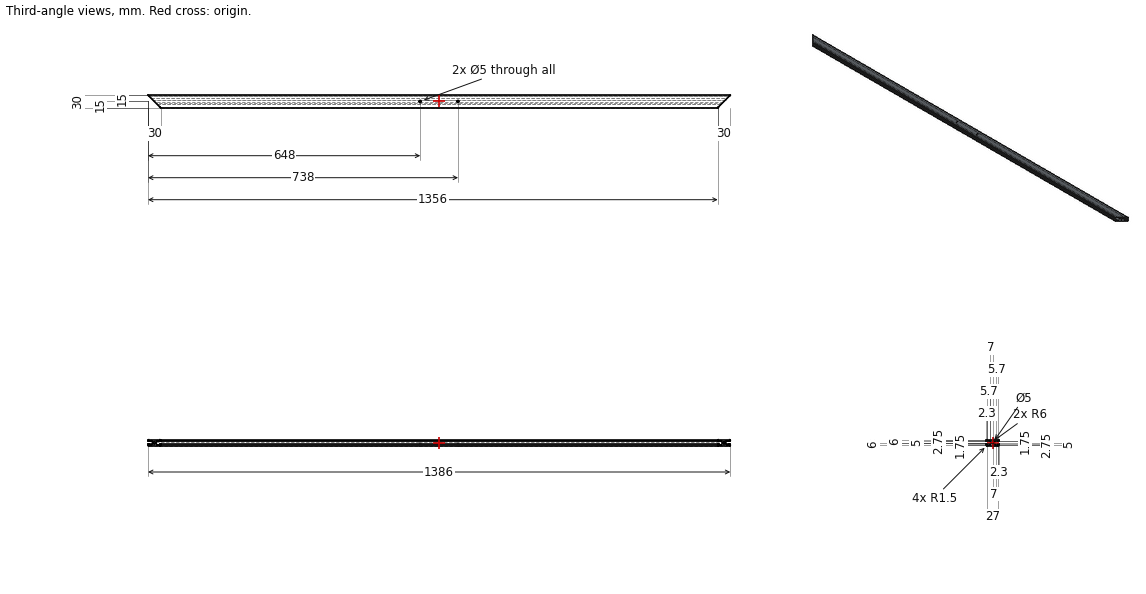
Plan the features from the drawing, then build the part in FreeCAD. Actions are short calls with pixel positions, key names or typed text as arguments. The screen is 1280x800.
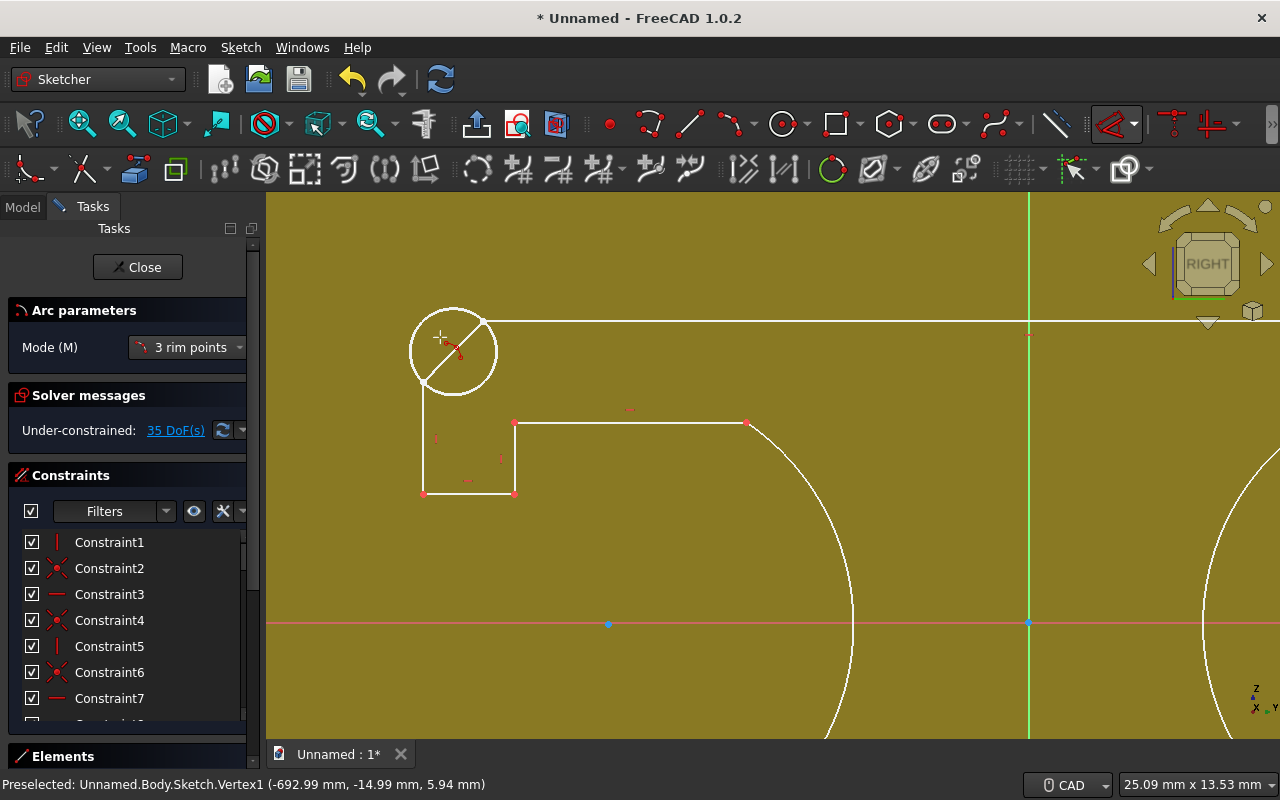
click(440, 337)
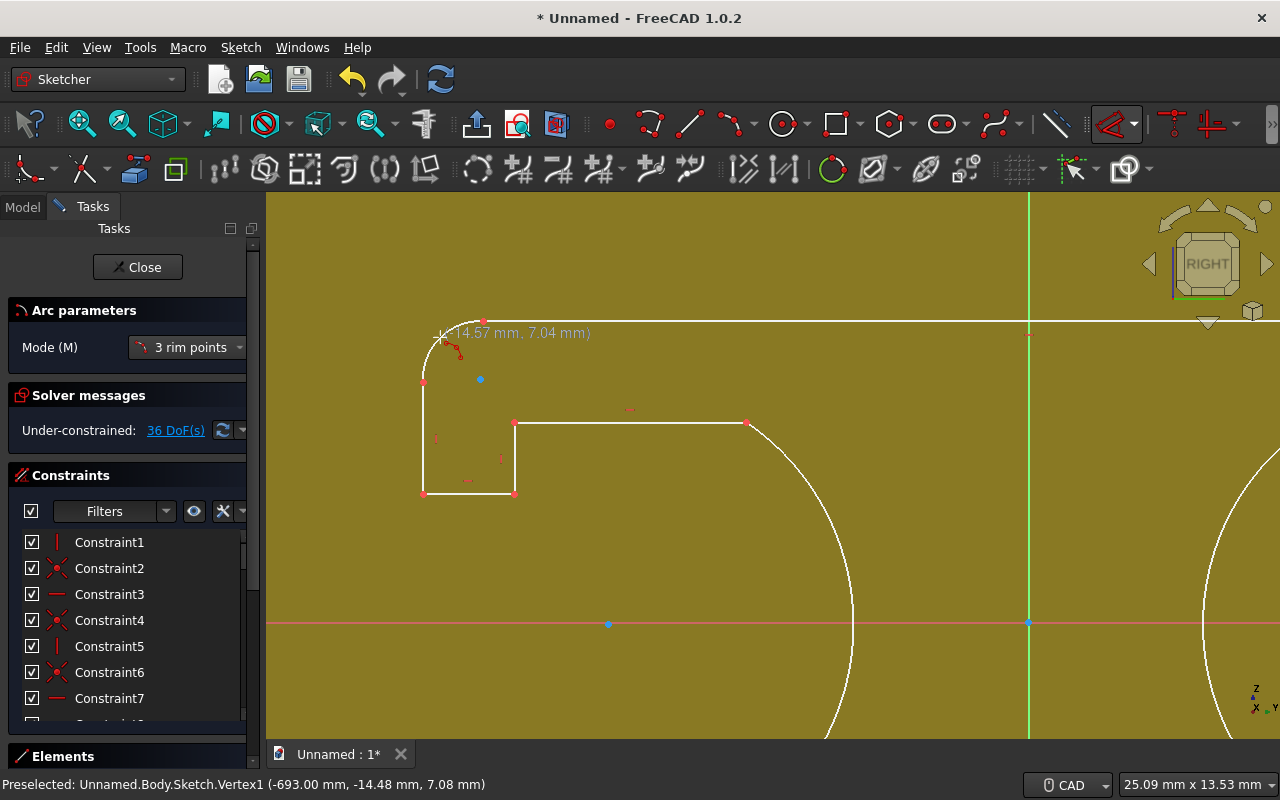
click(784, 124)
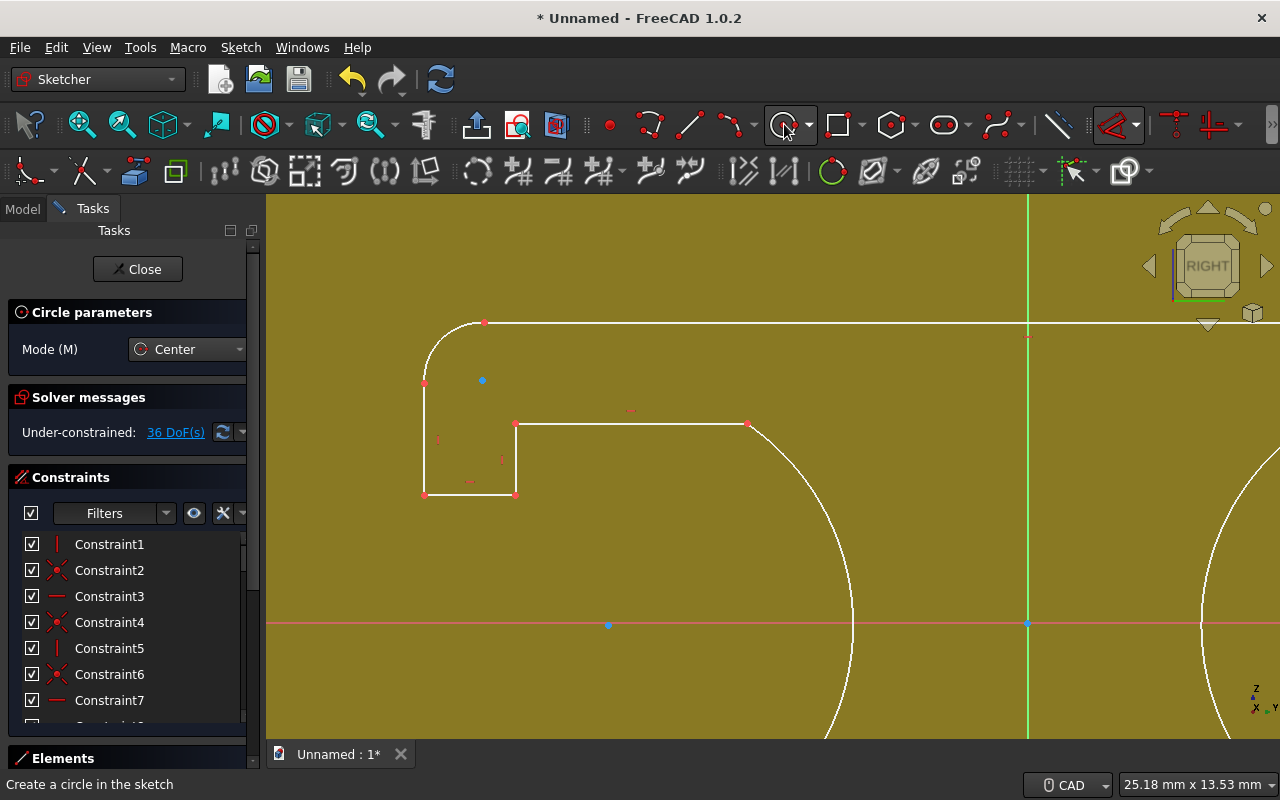
click(1028, 623)
click(1099, 552)
key(Escape)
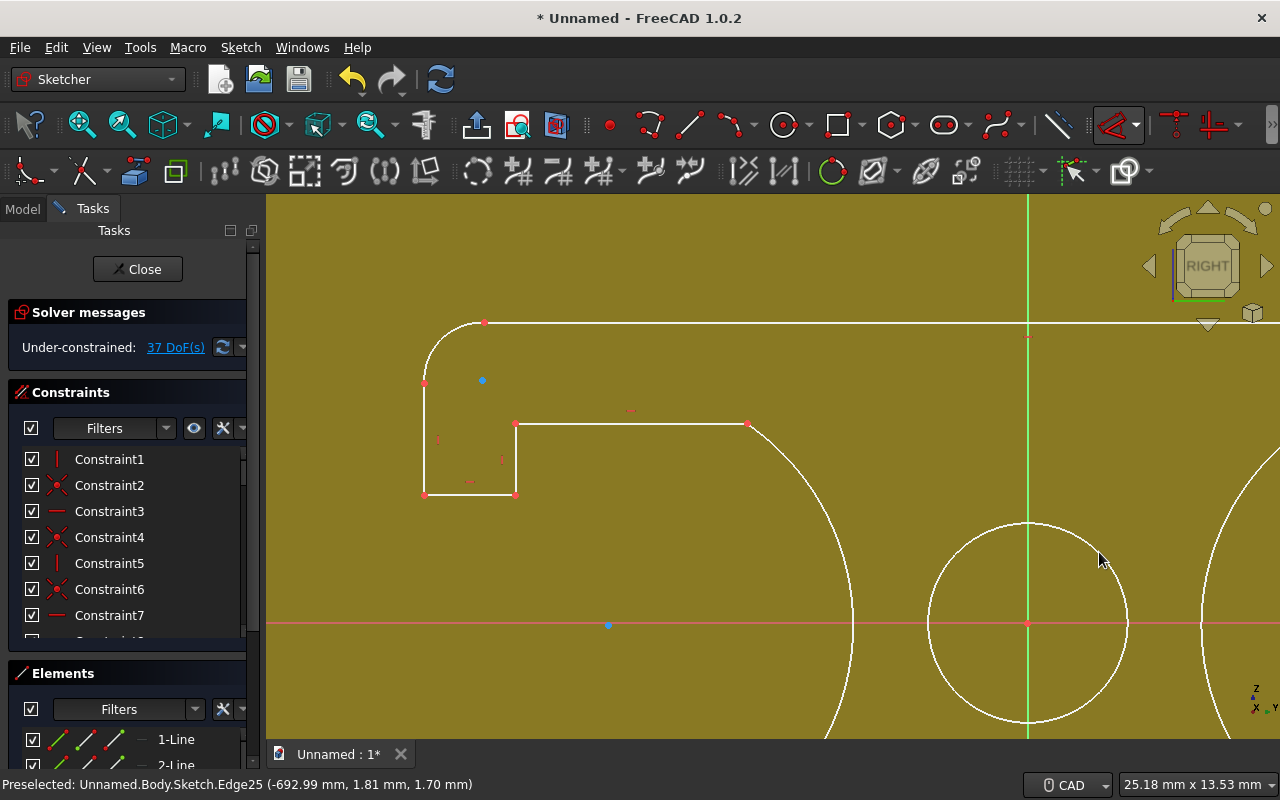
click(424, 417)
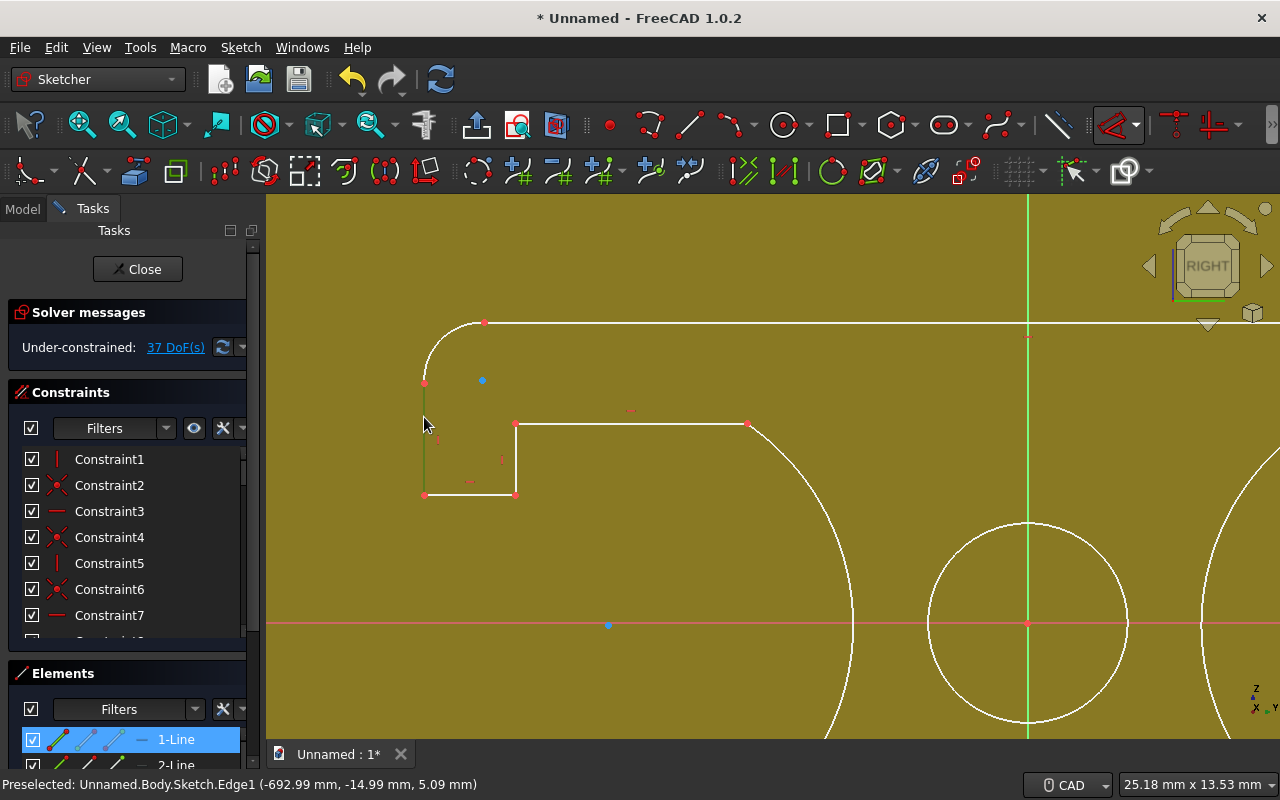
click(457, 328)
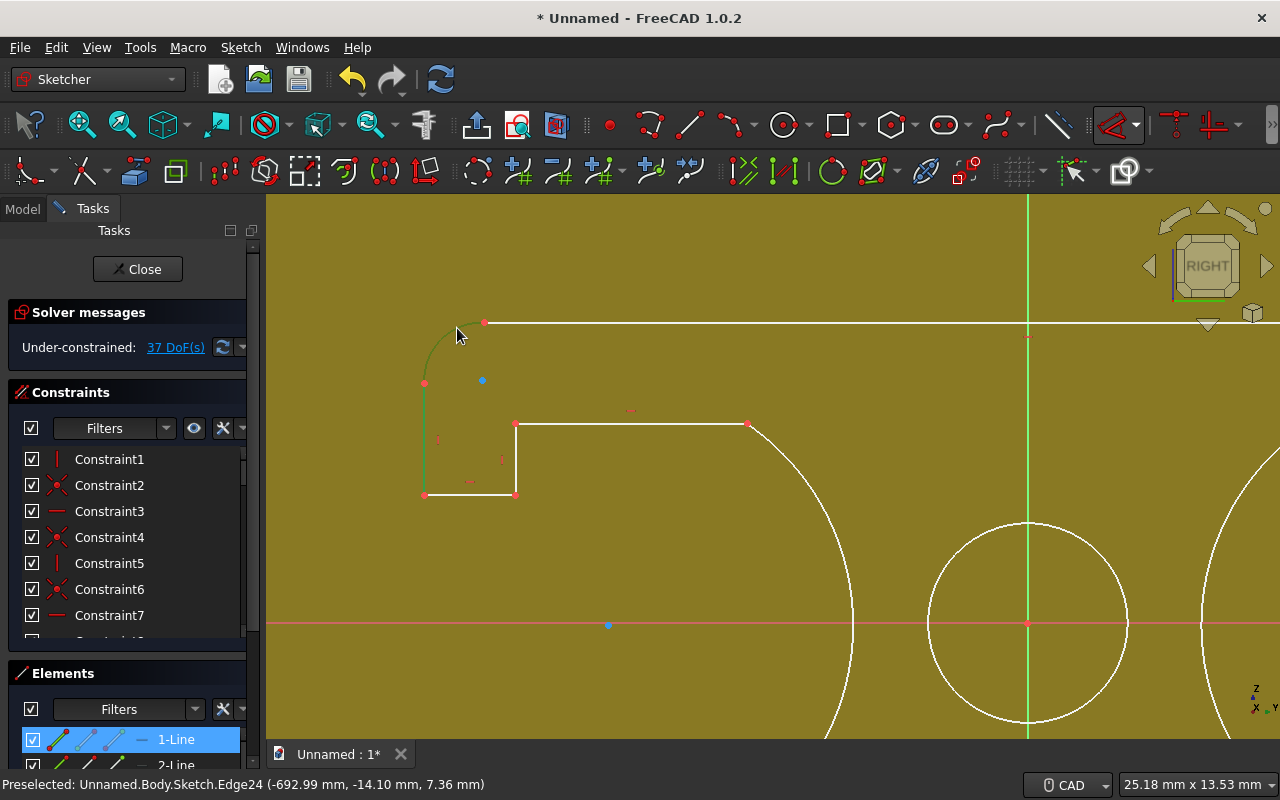
key(t)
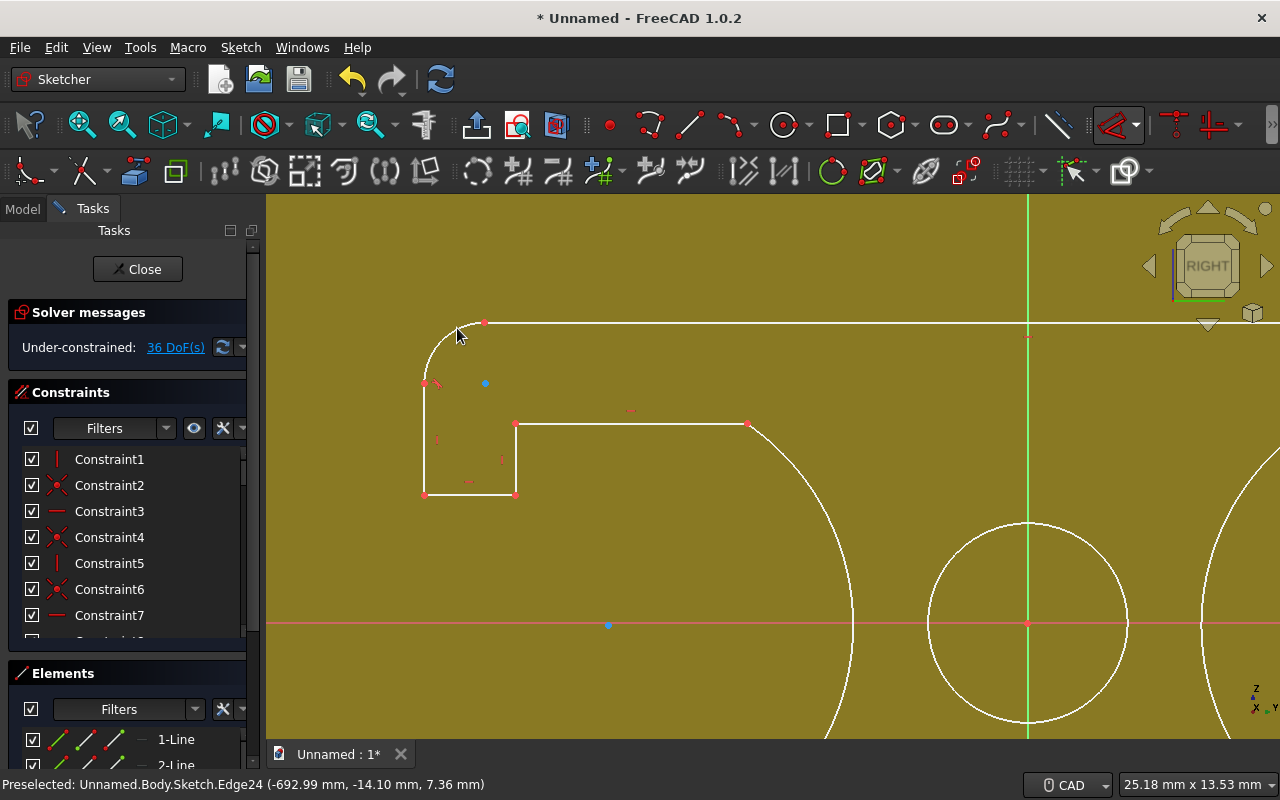
scroll(441, 339, down, 4)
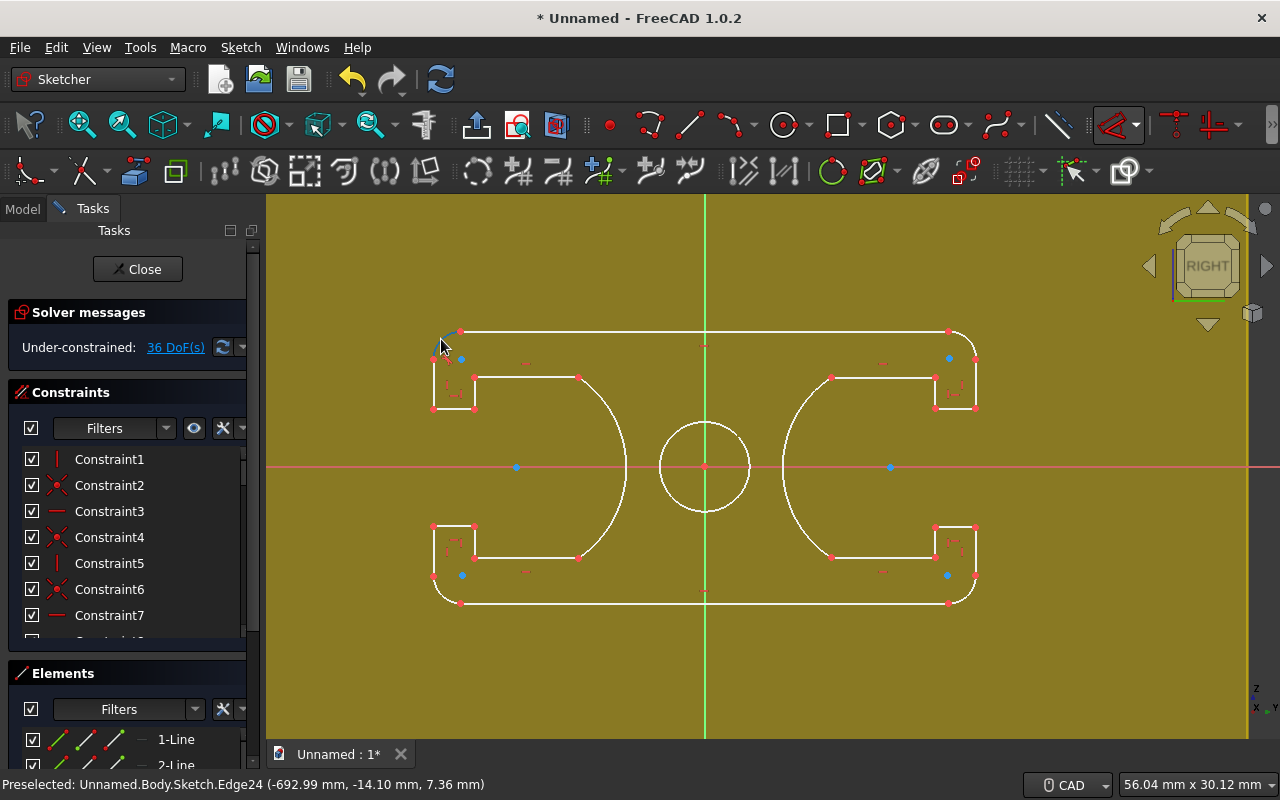
click(434, 541)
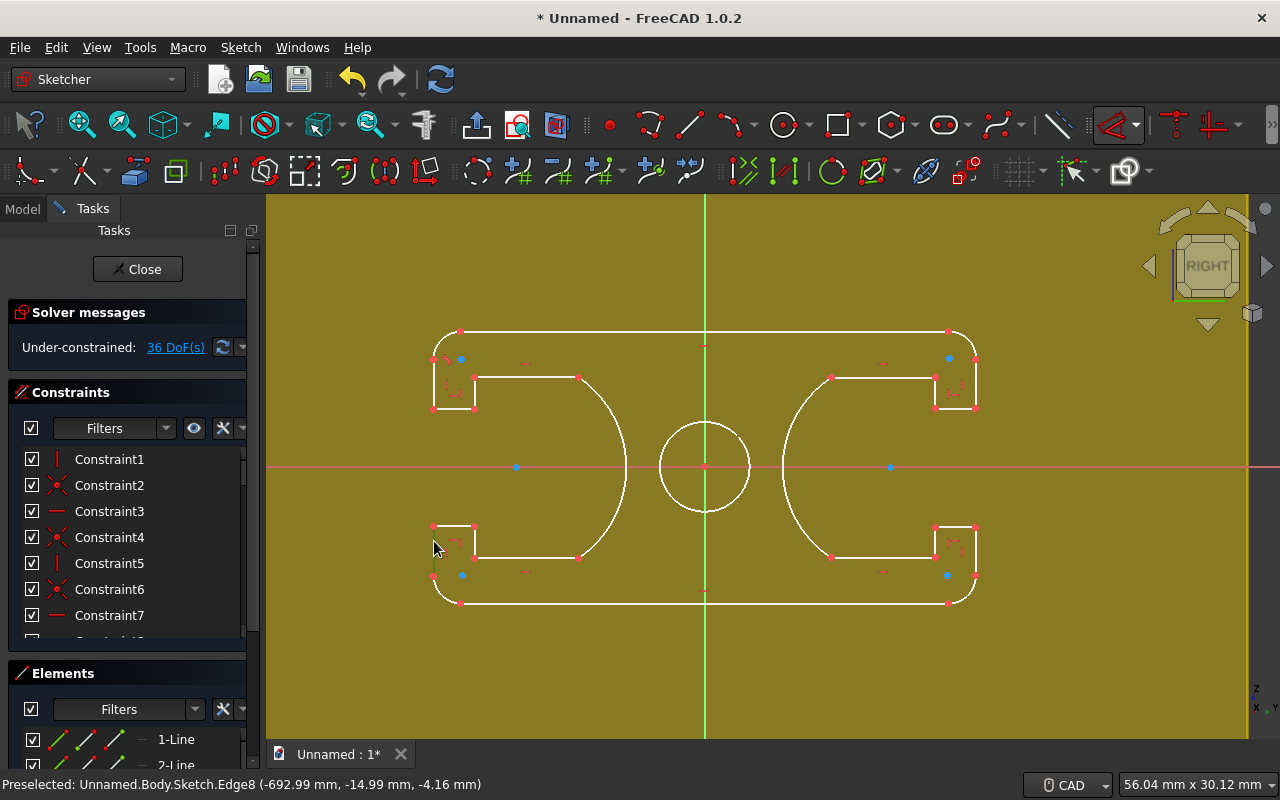
click(437, 588)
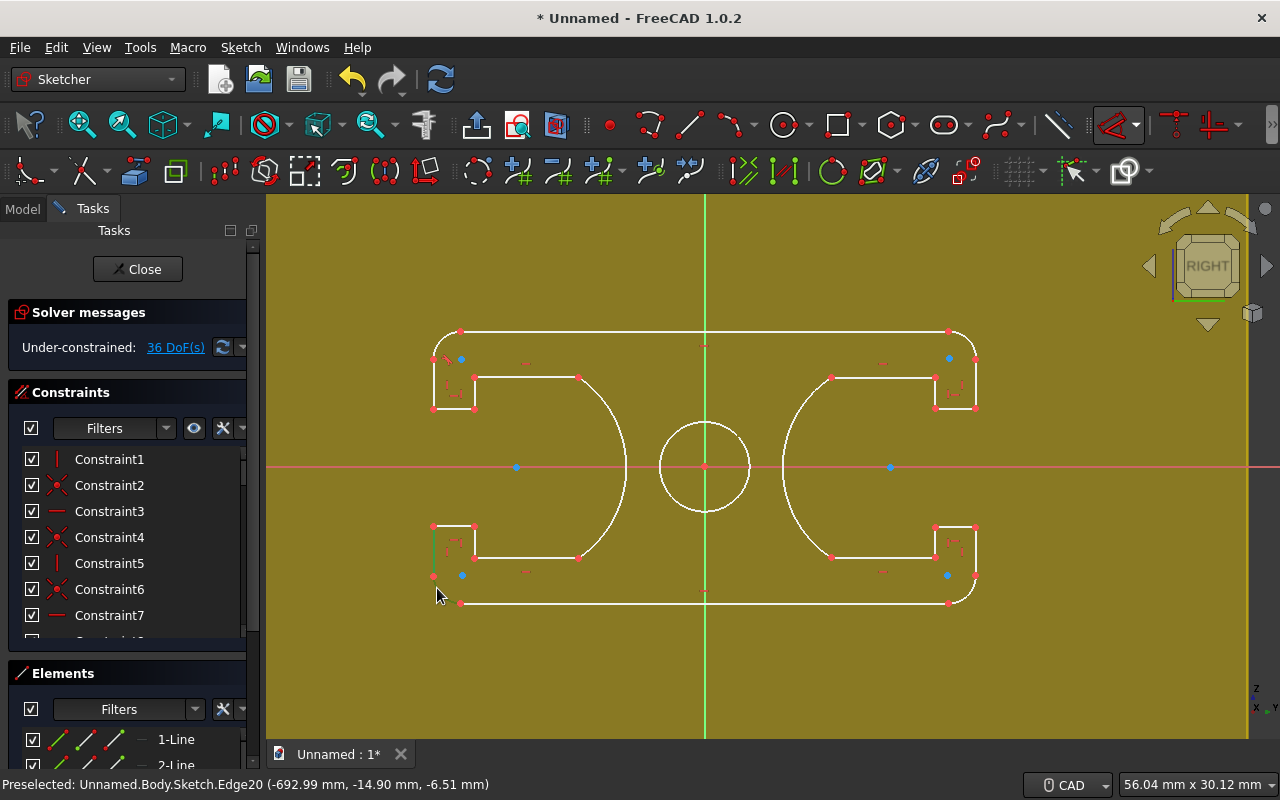
key(t)